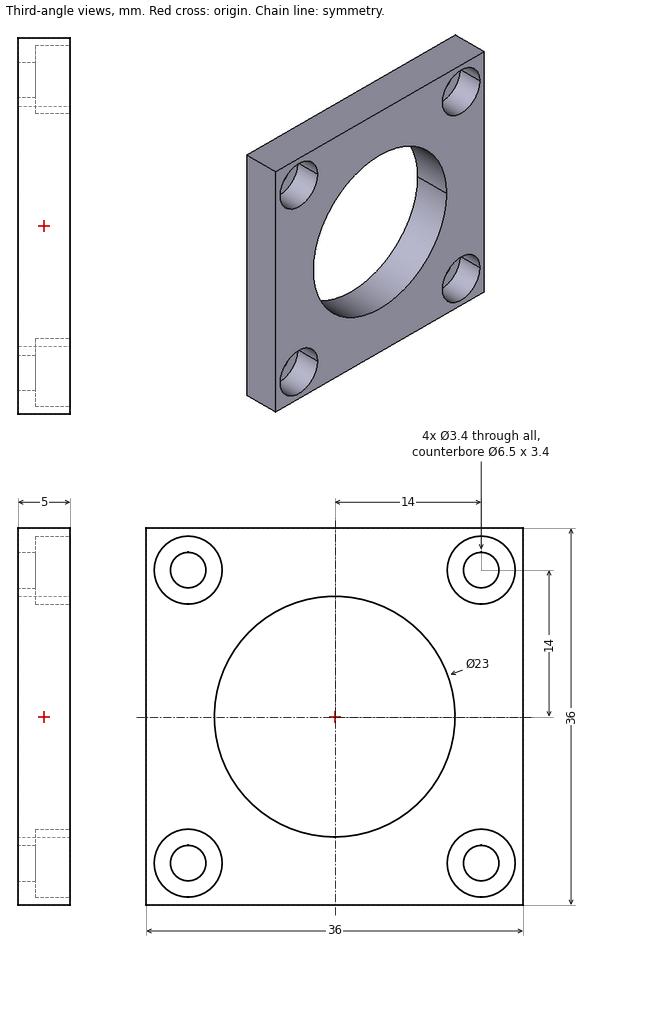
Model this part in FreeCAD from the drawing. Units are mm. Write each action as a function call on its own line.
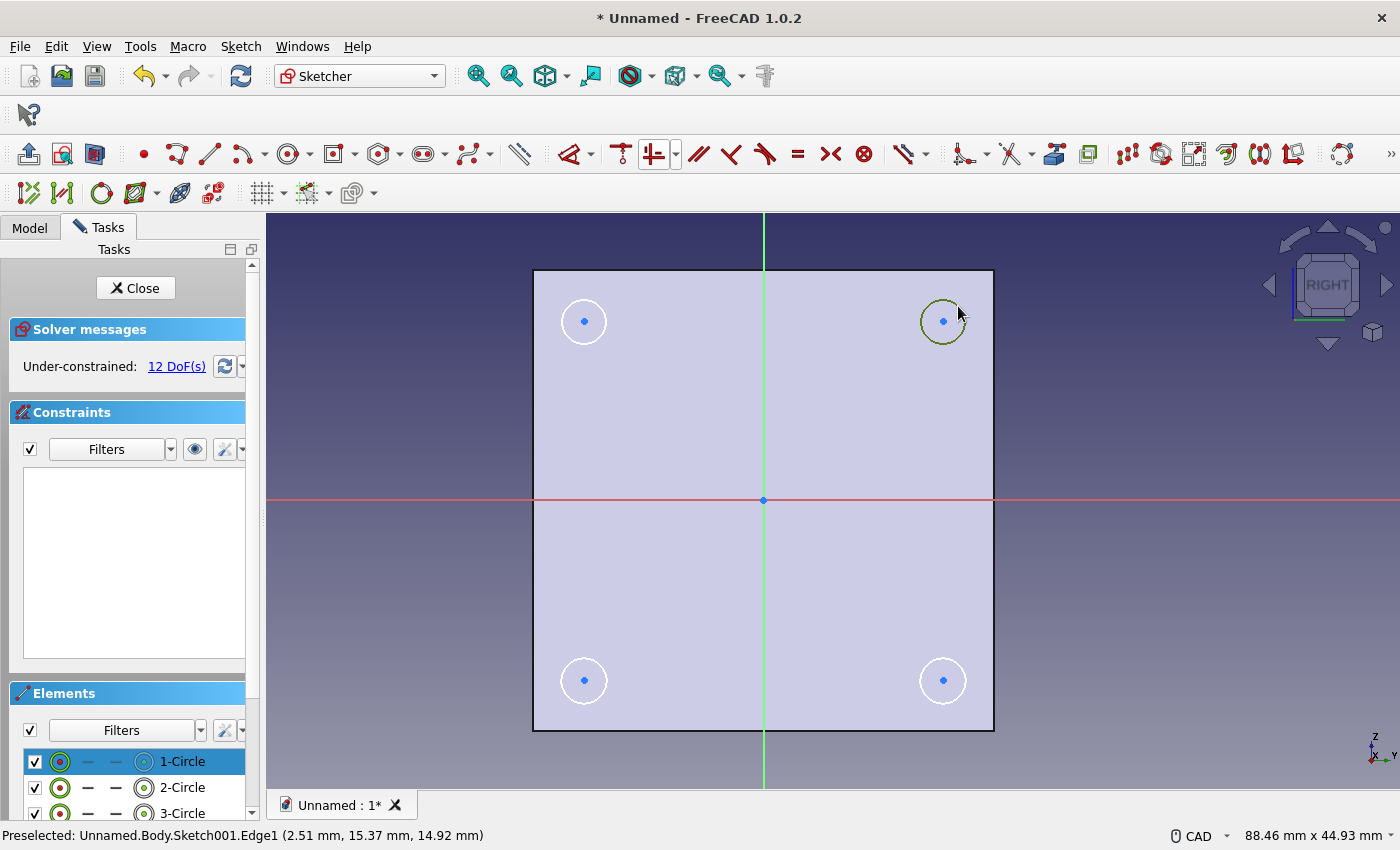
click(959, 665)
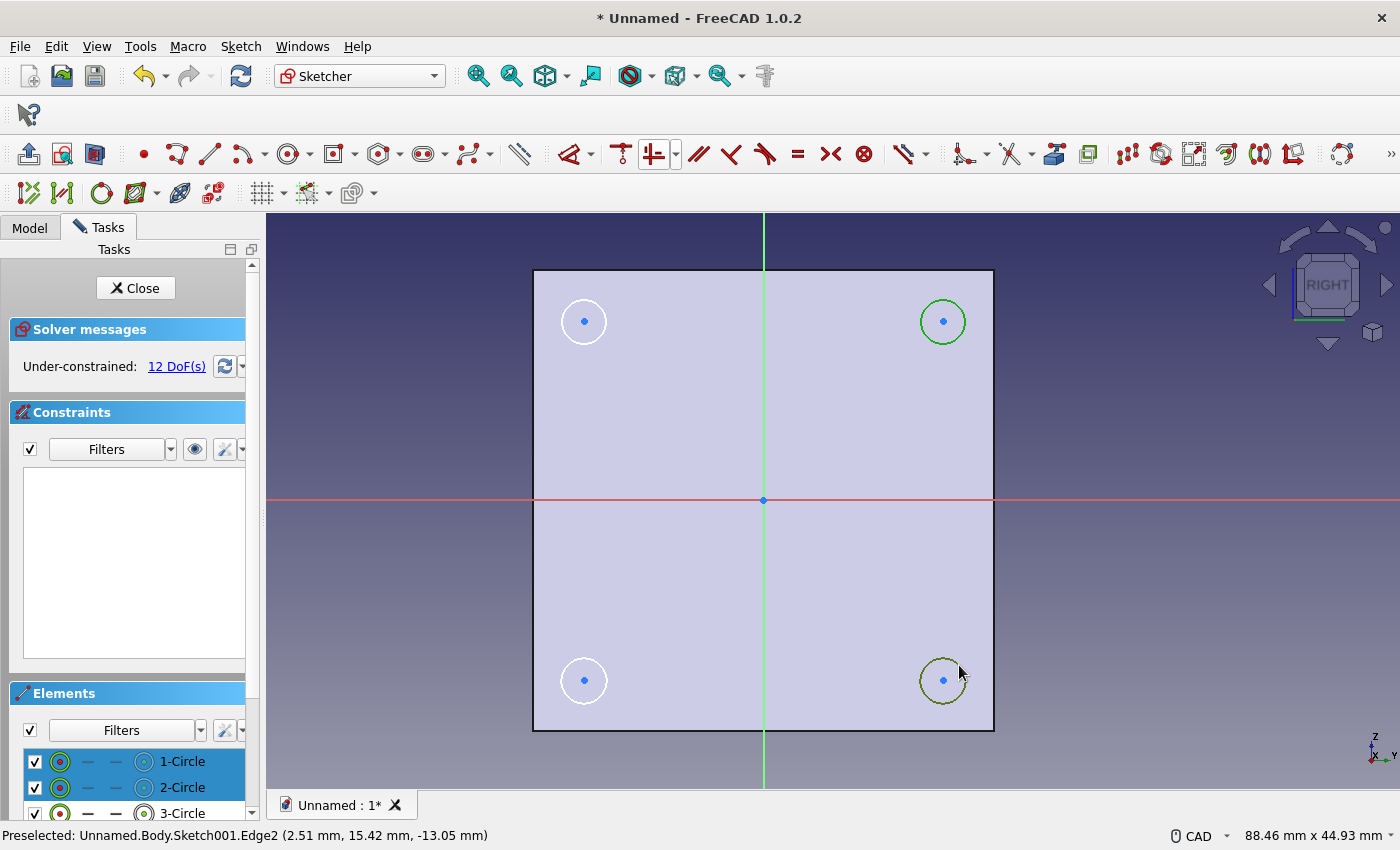
click(599, 306)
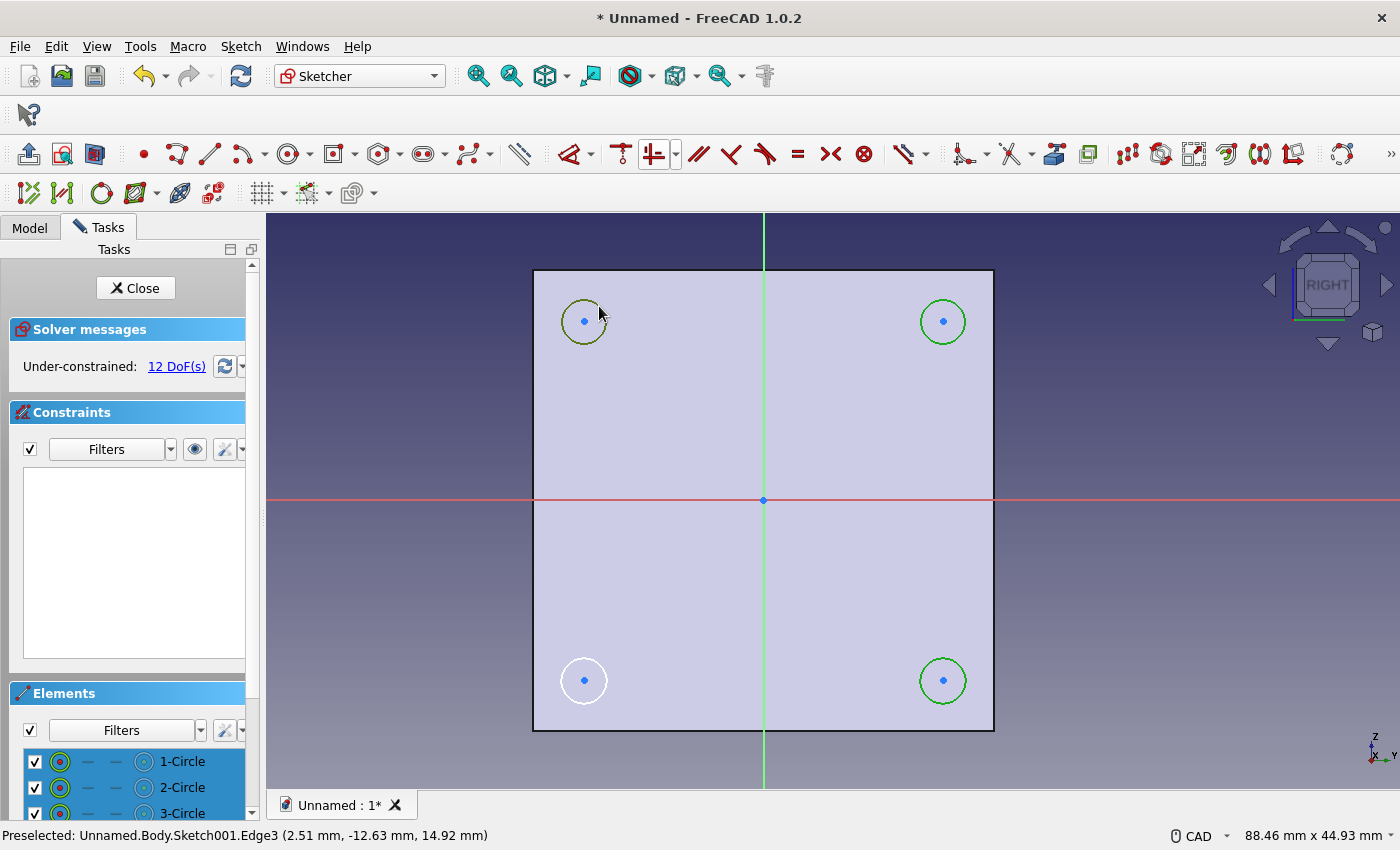
click(600, 665)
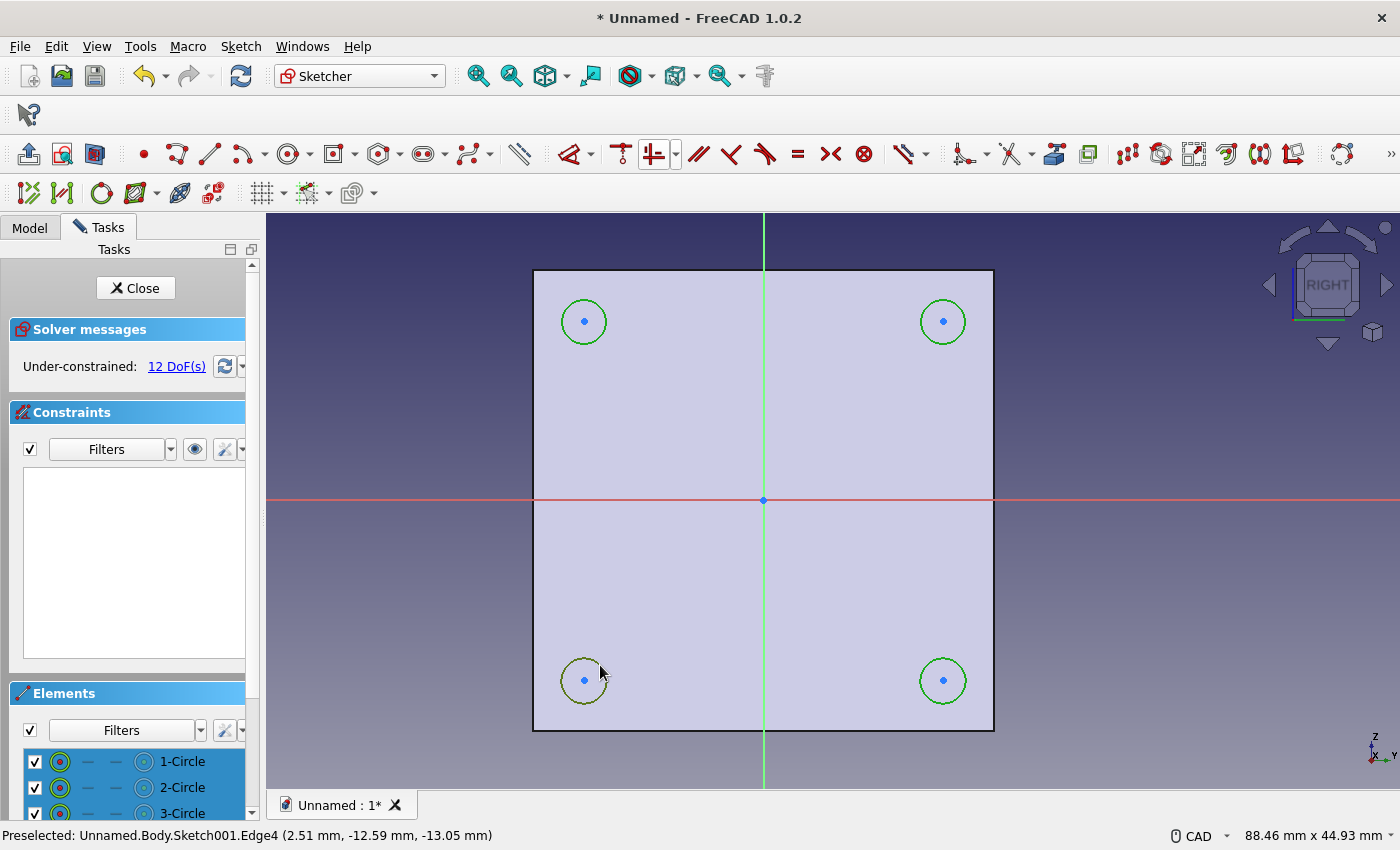
click(798, 154)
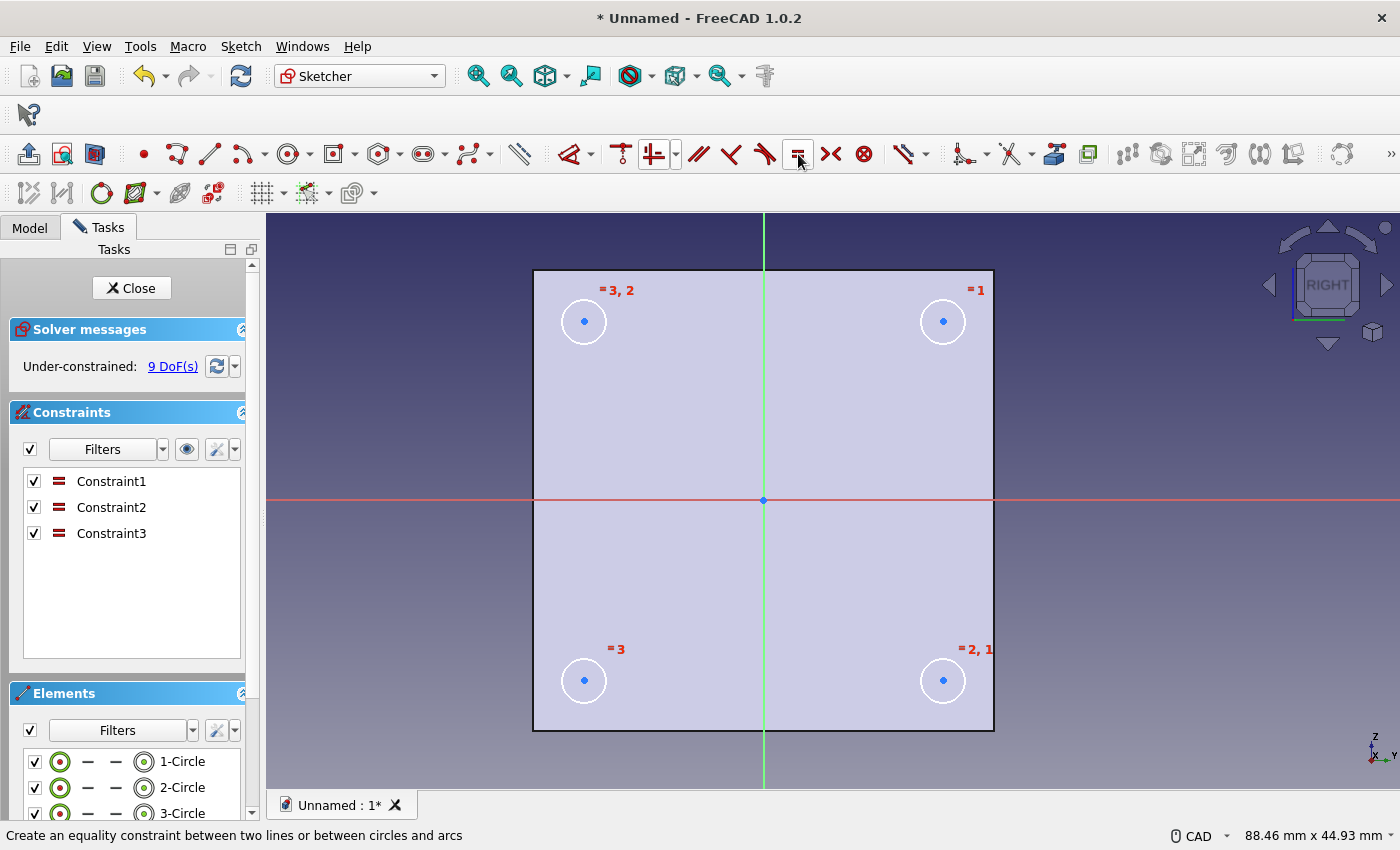
click(943, 322)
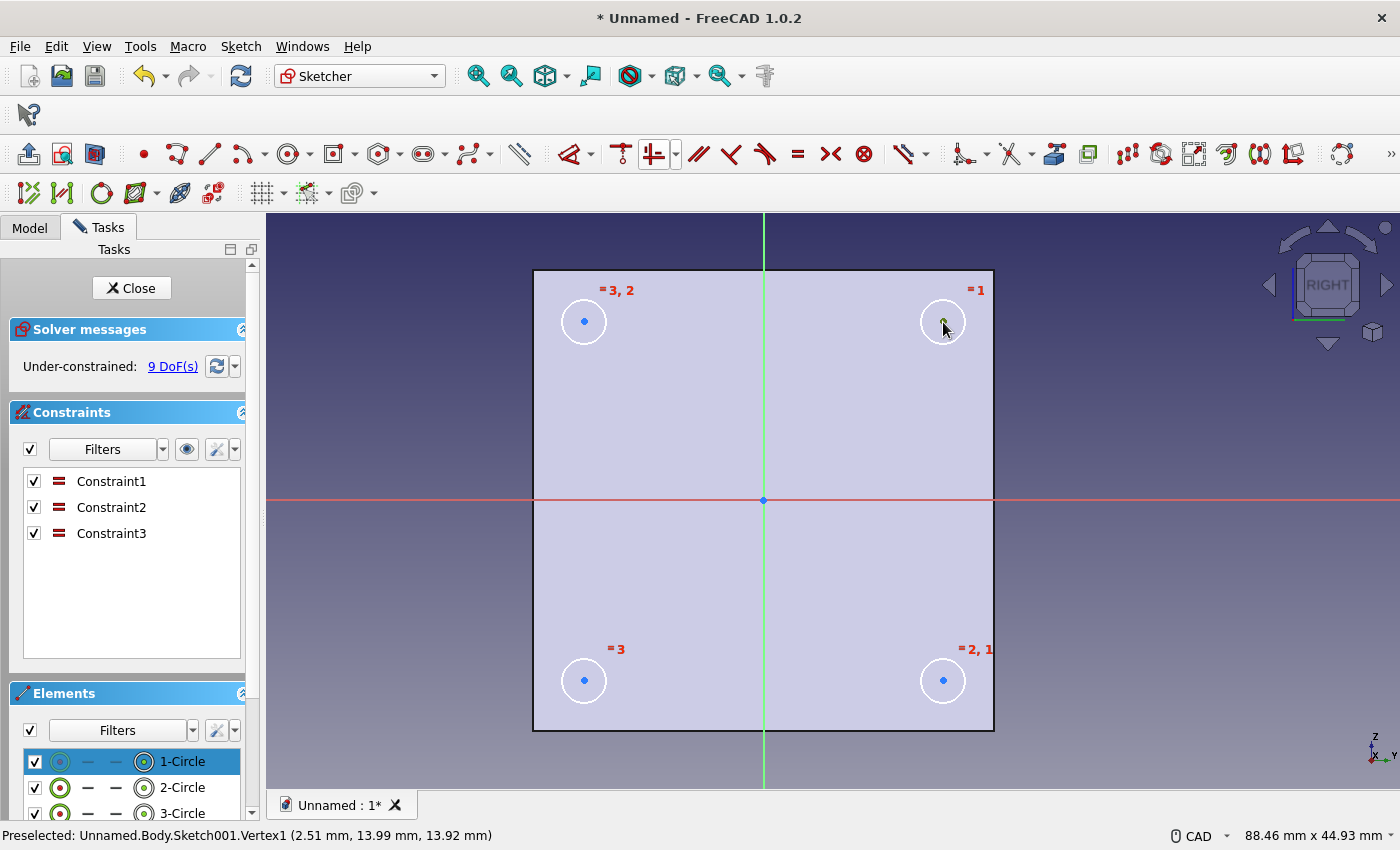
click(943, 681)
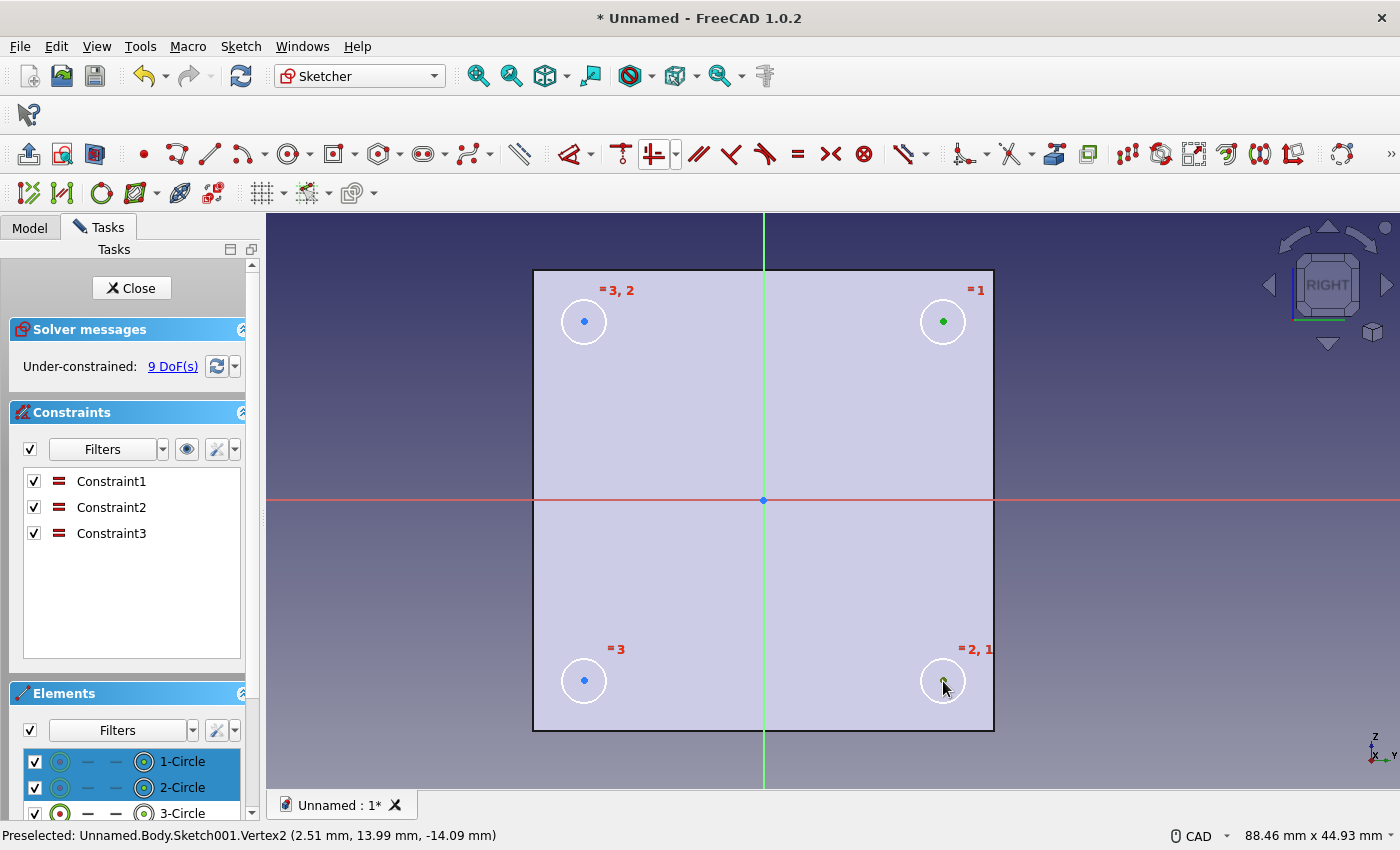
click(361, 500)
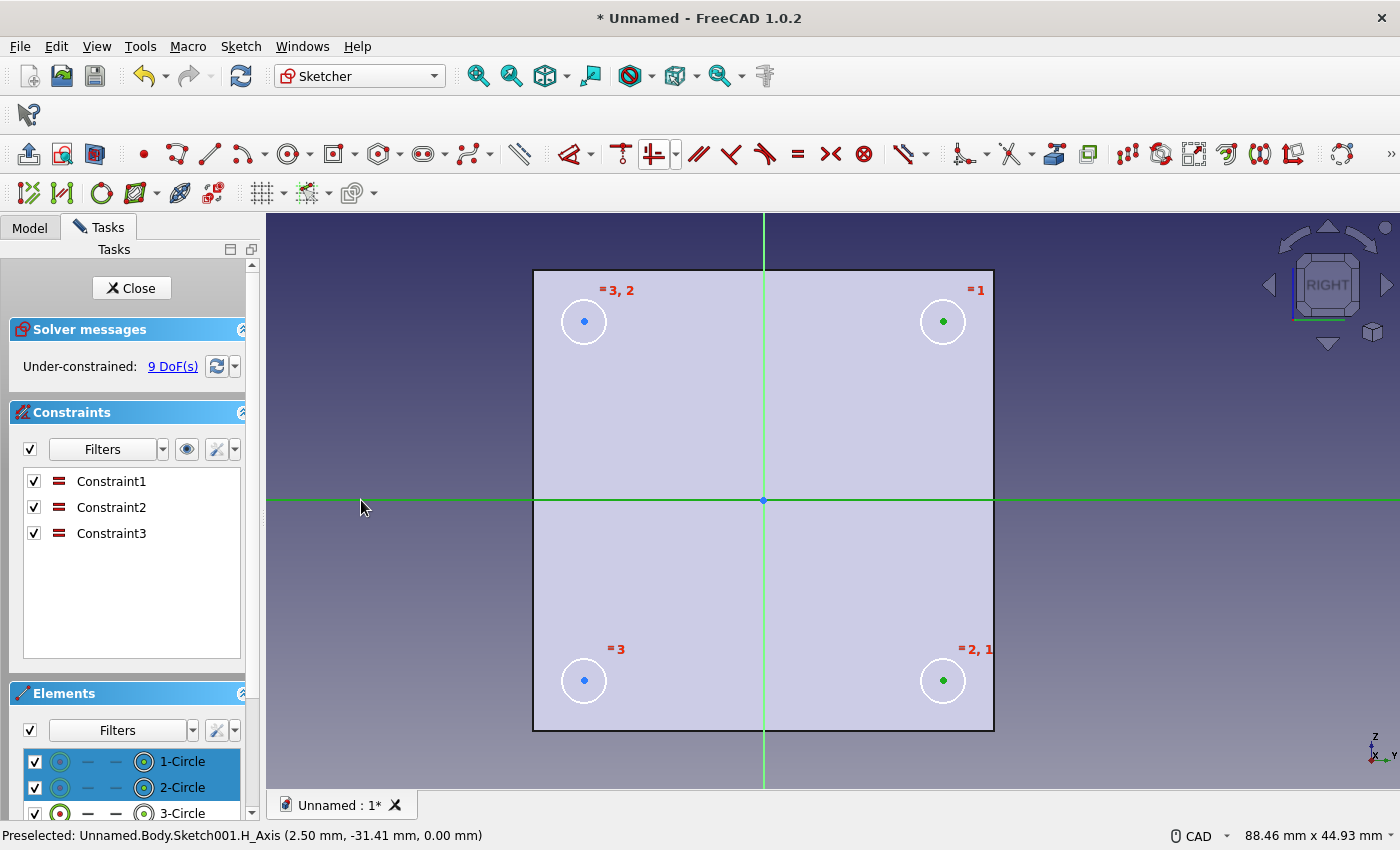
click(831, 154)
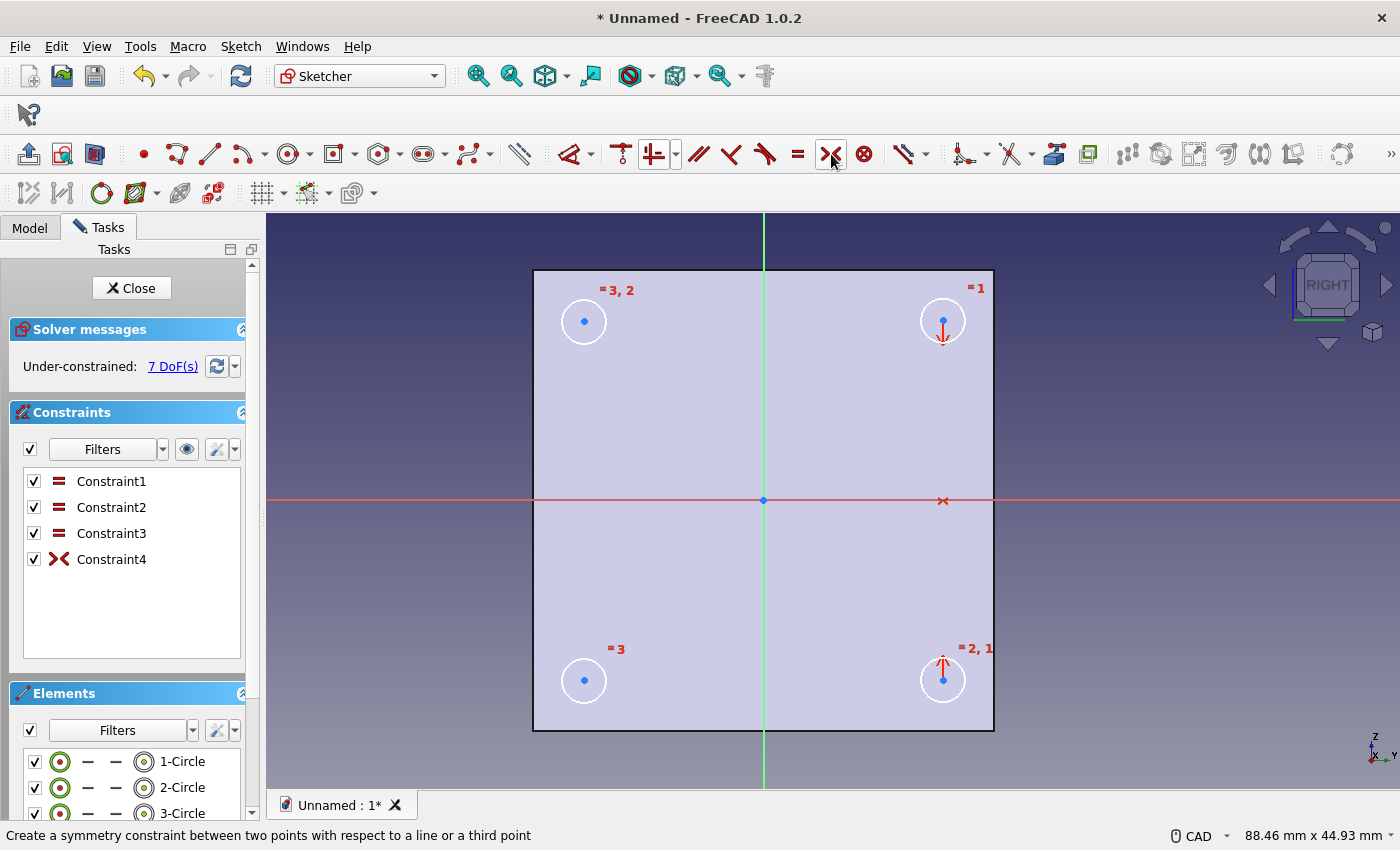
click(943, 321)